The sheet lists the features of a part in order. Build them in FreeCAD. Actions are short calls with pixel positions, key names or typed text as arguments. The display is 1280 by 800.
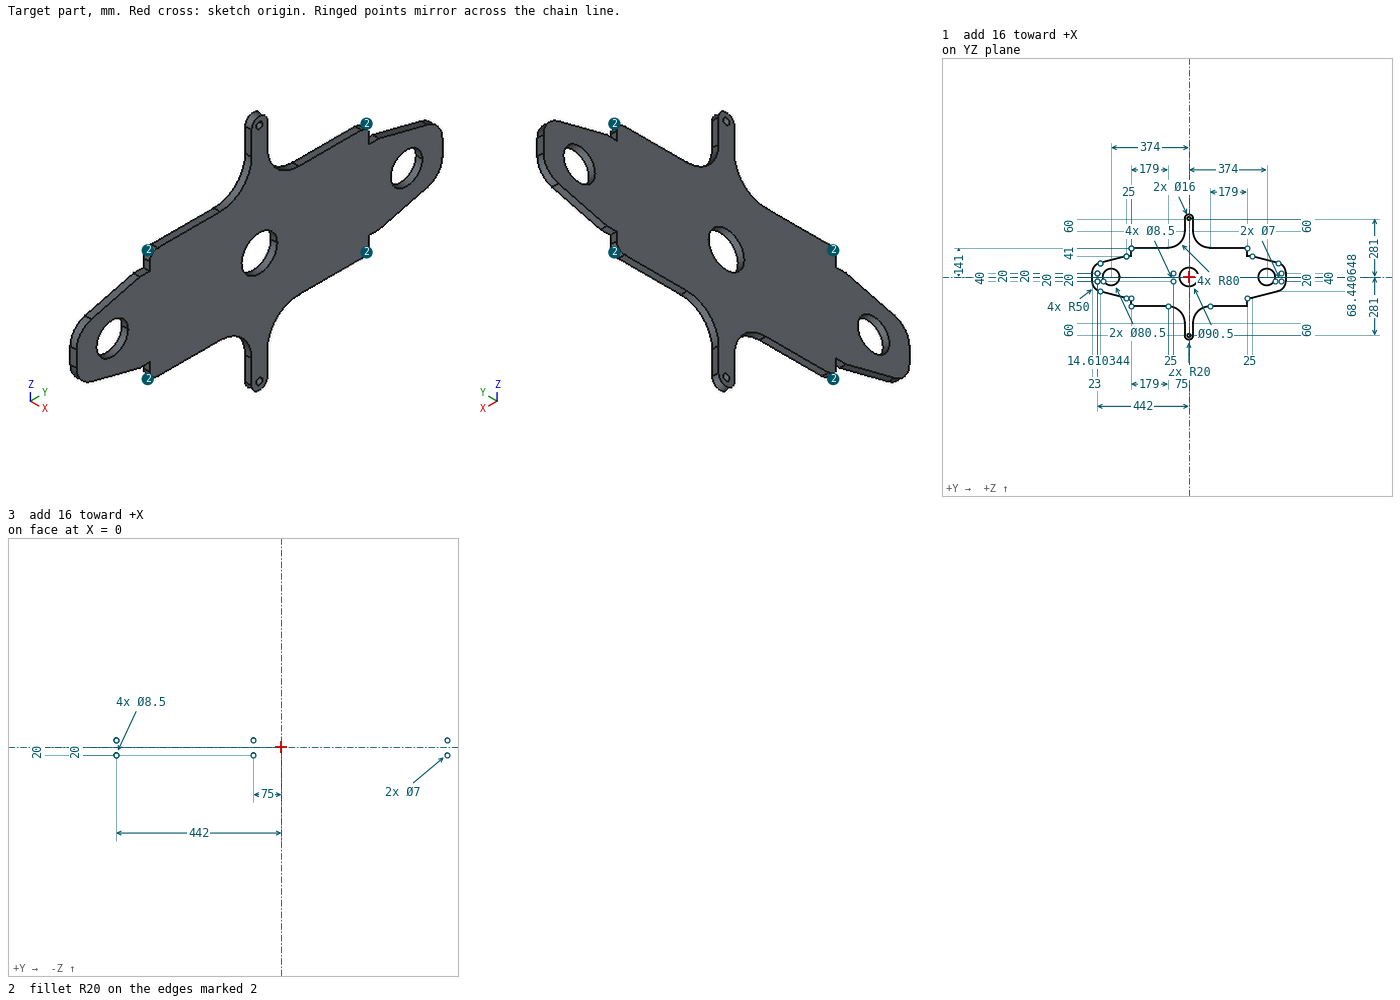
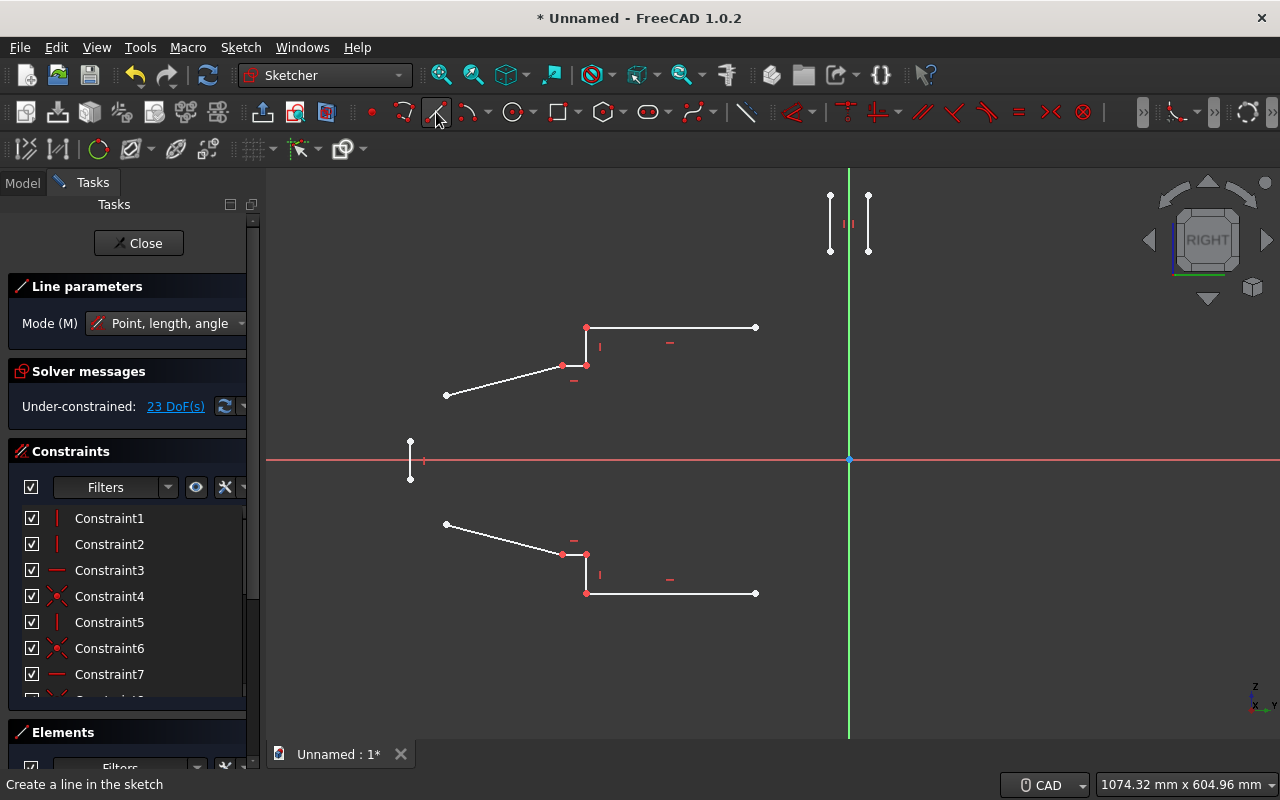
click(831, 668)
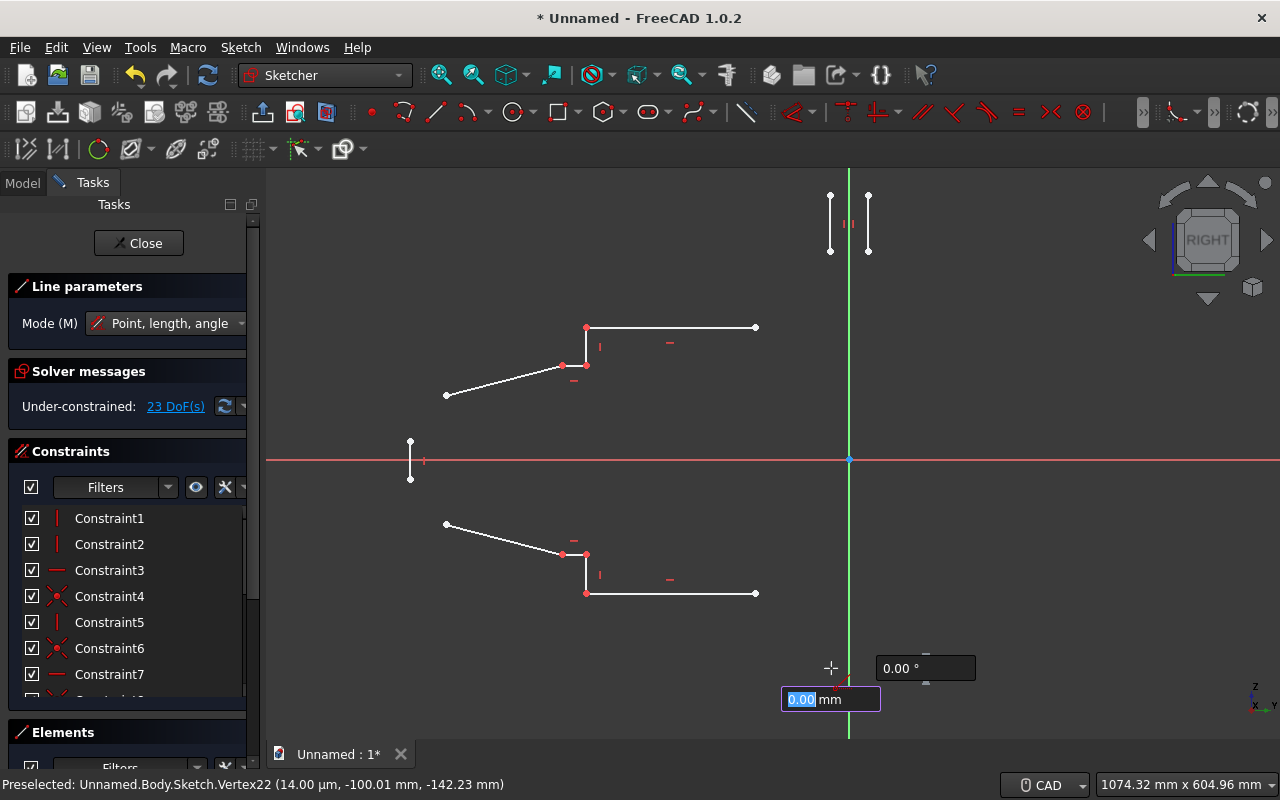
scroll(410, 441, down, 2)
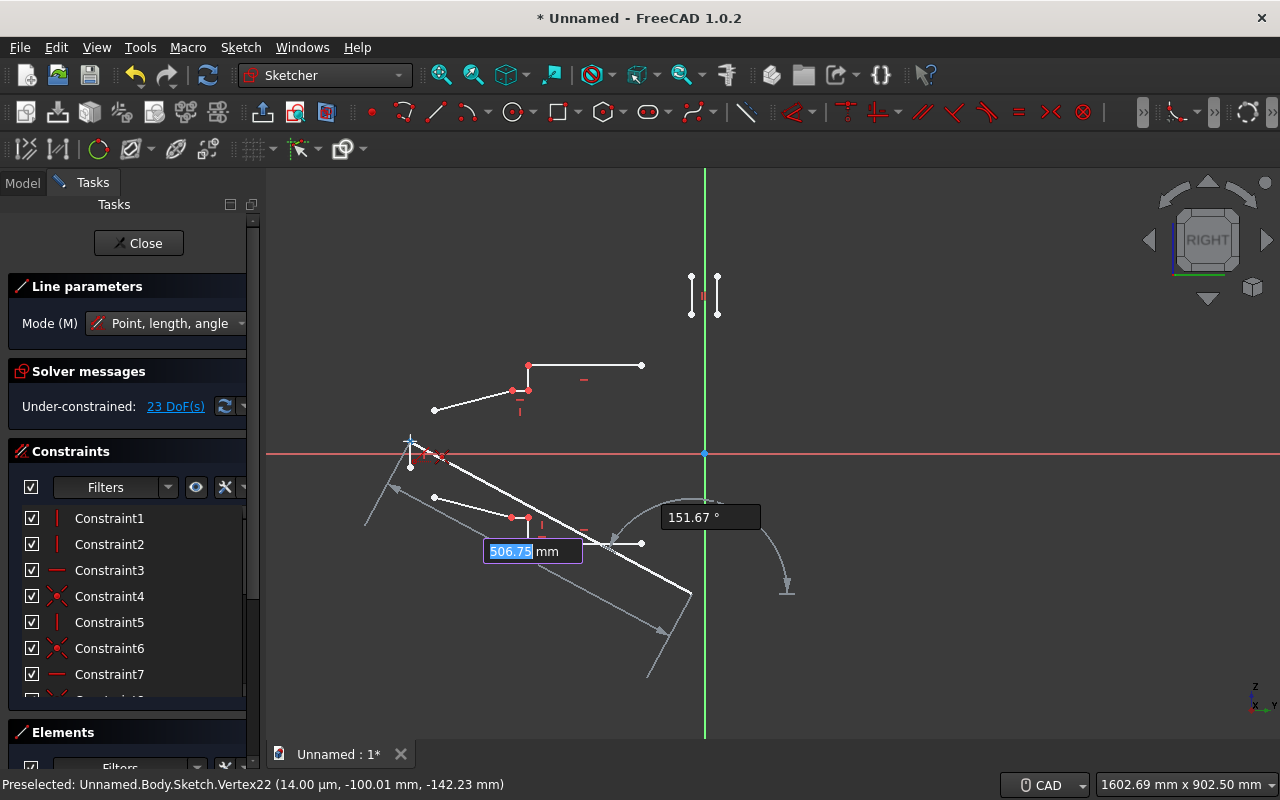
scroll(692, 632, up, 2)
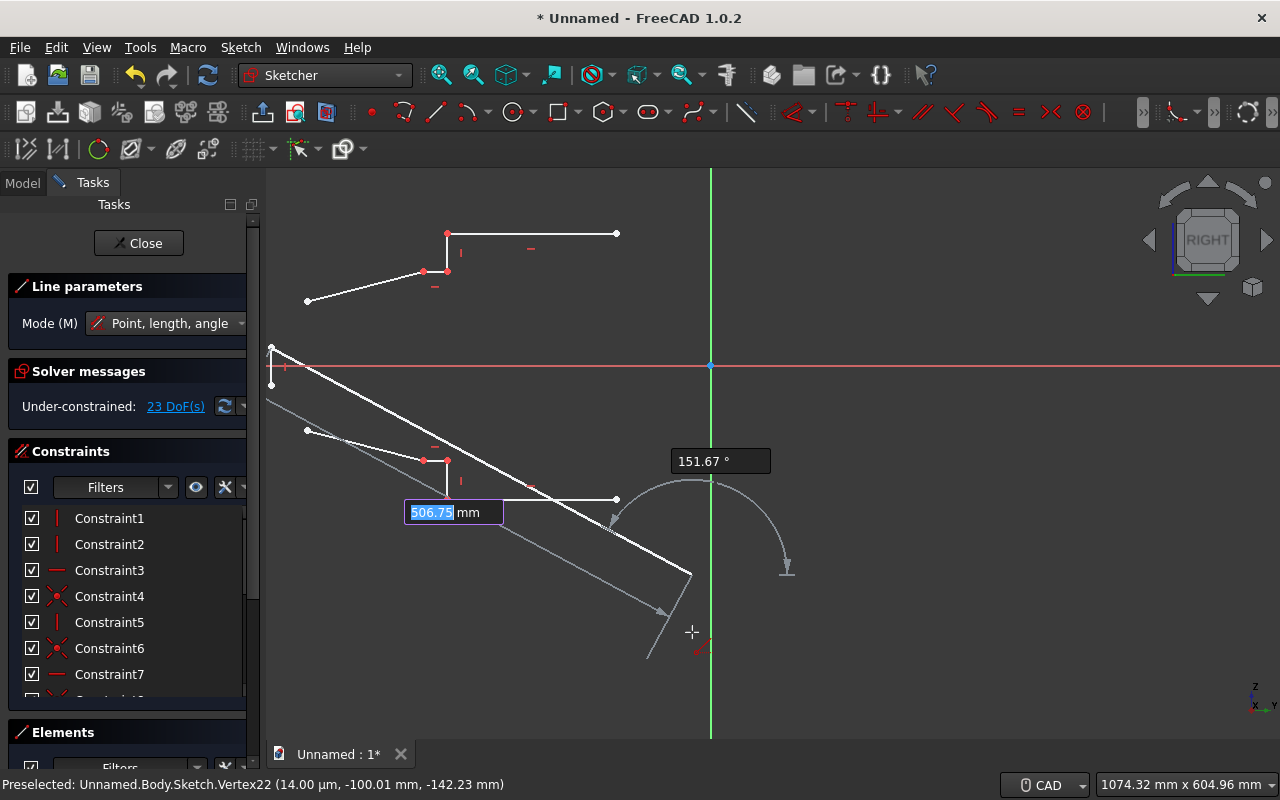
click(692, 631)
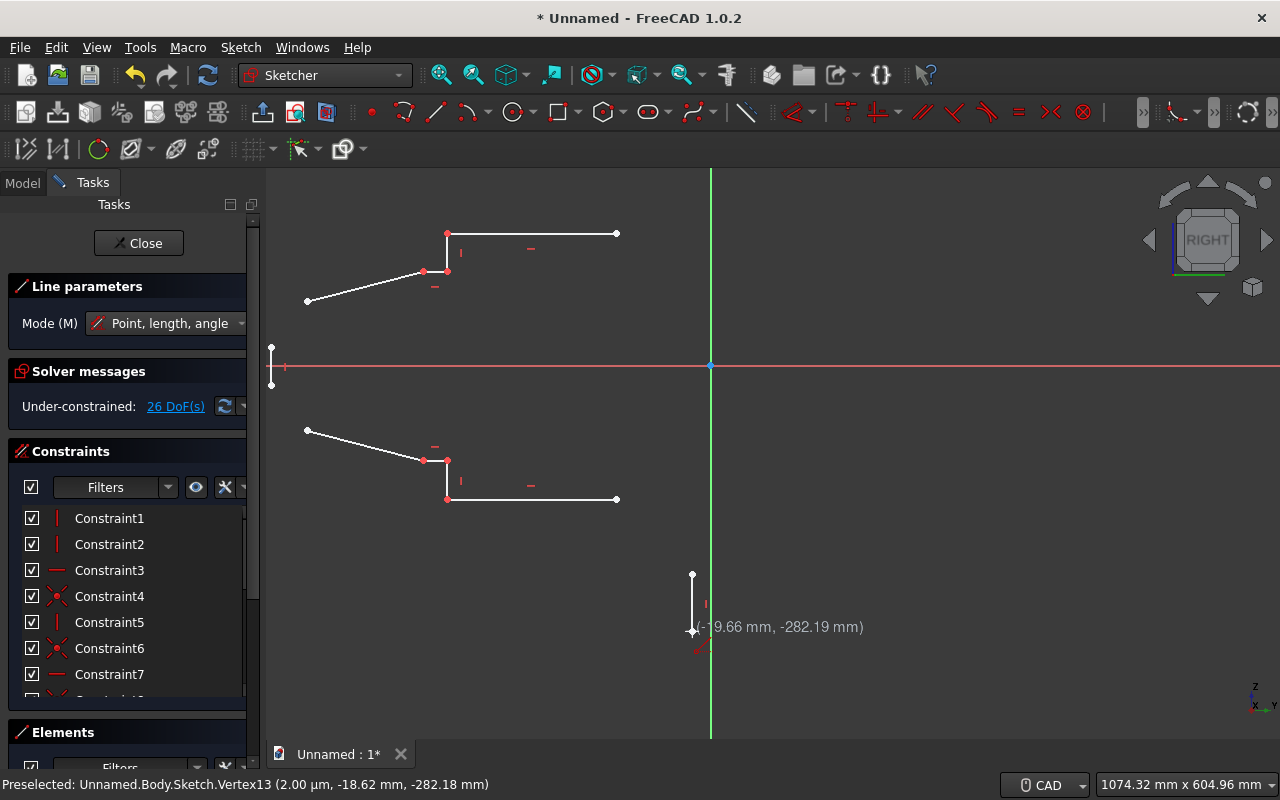
click(729, 631)
click(729, 574)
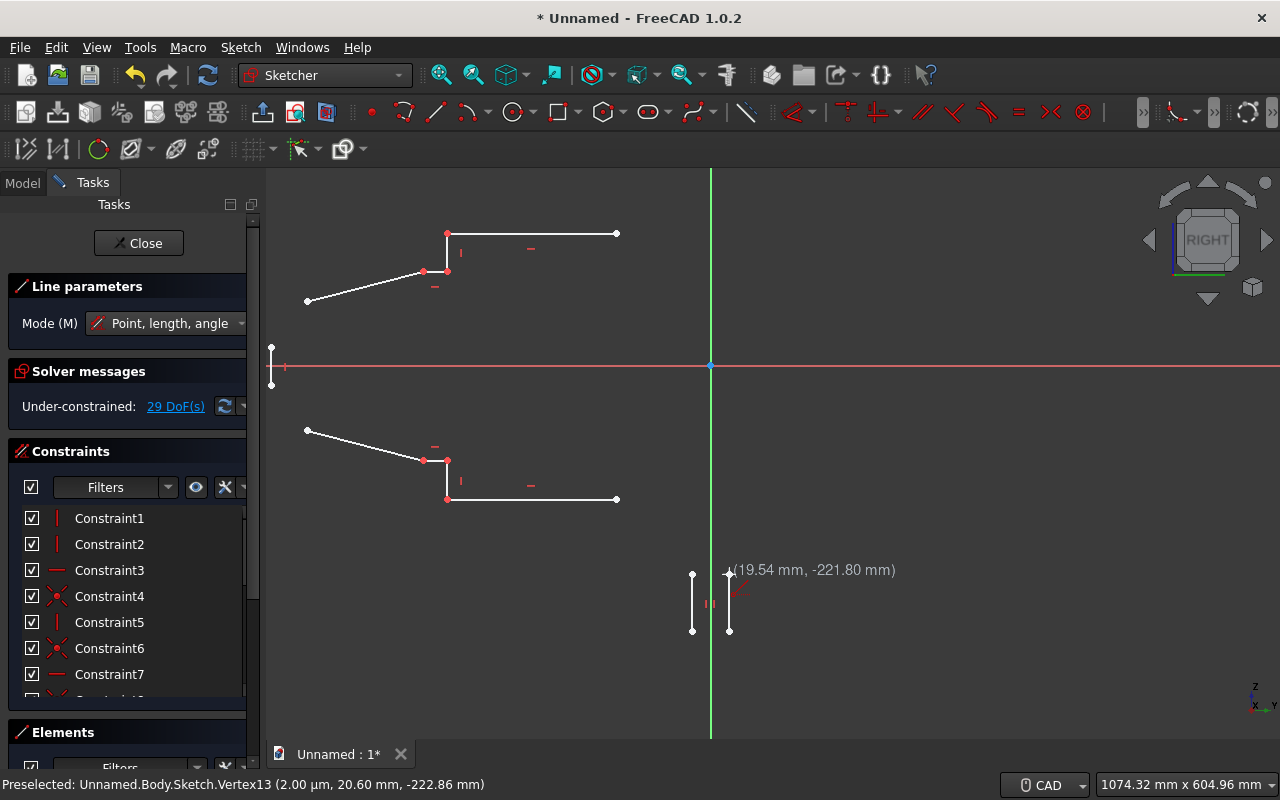
click(404, 112)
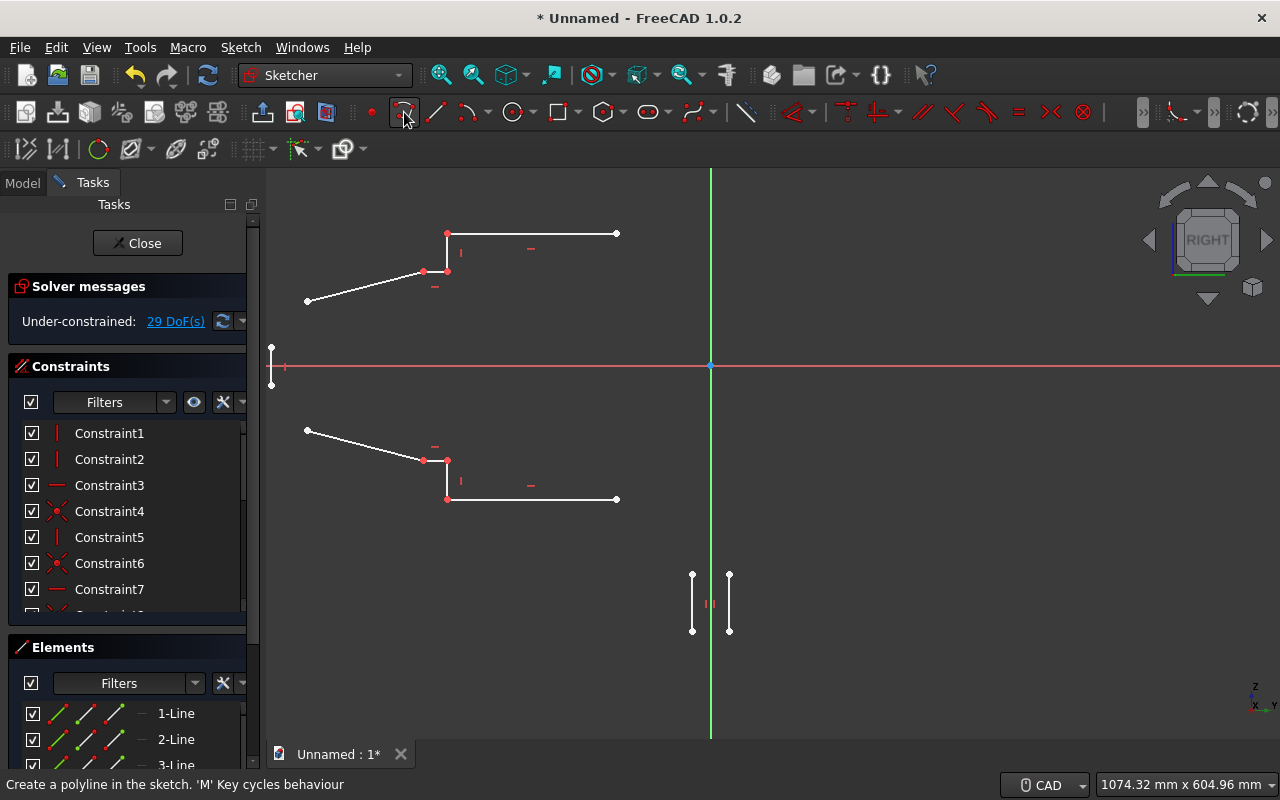
click(805, 499)
click(974, 499)
click(974, 460)
click(997, 460)
click(1114, 430)
right_click(1114, 430)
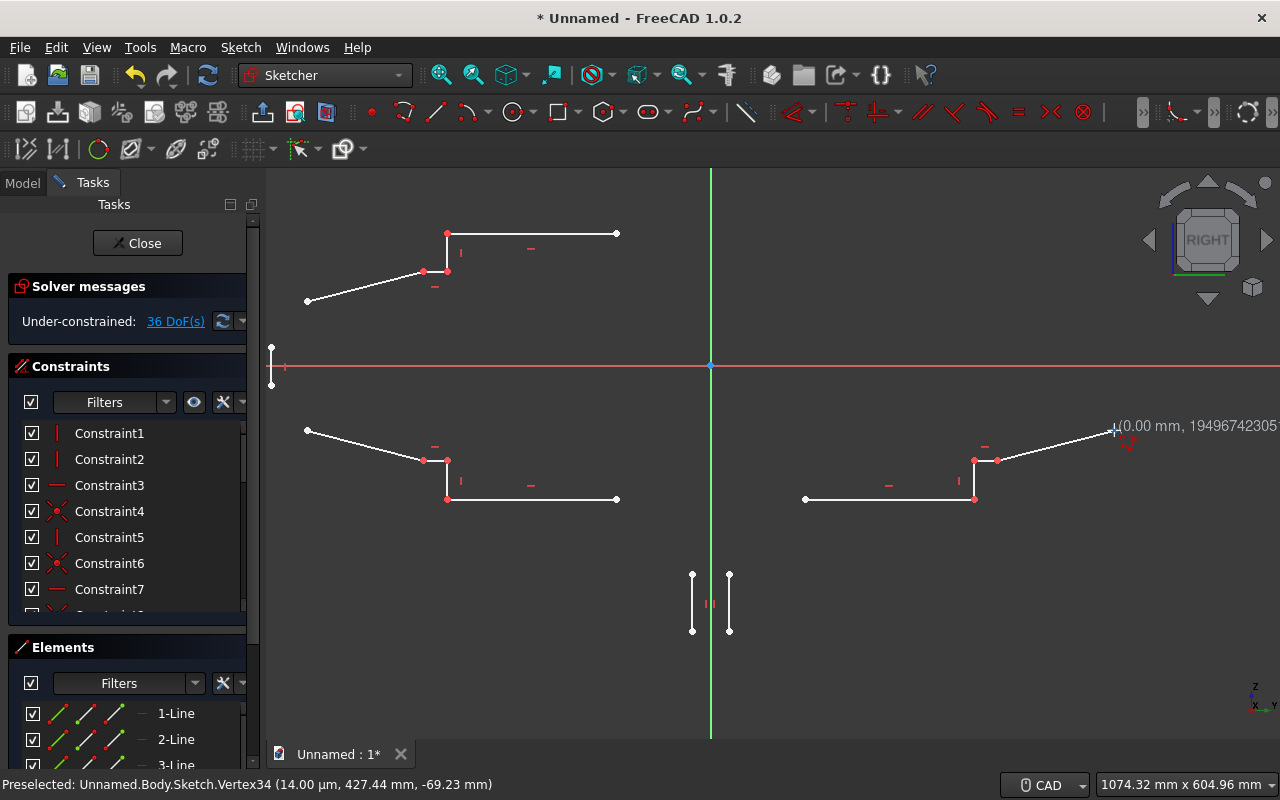
click(436, 112)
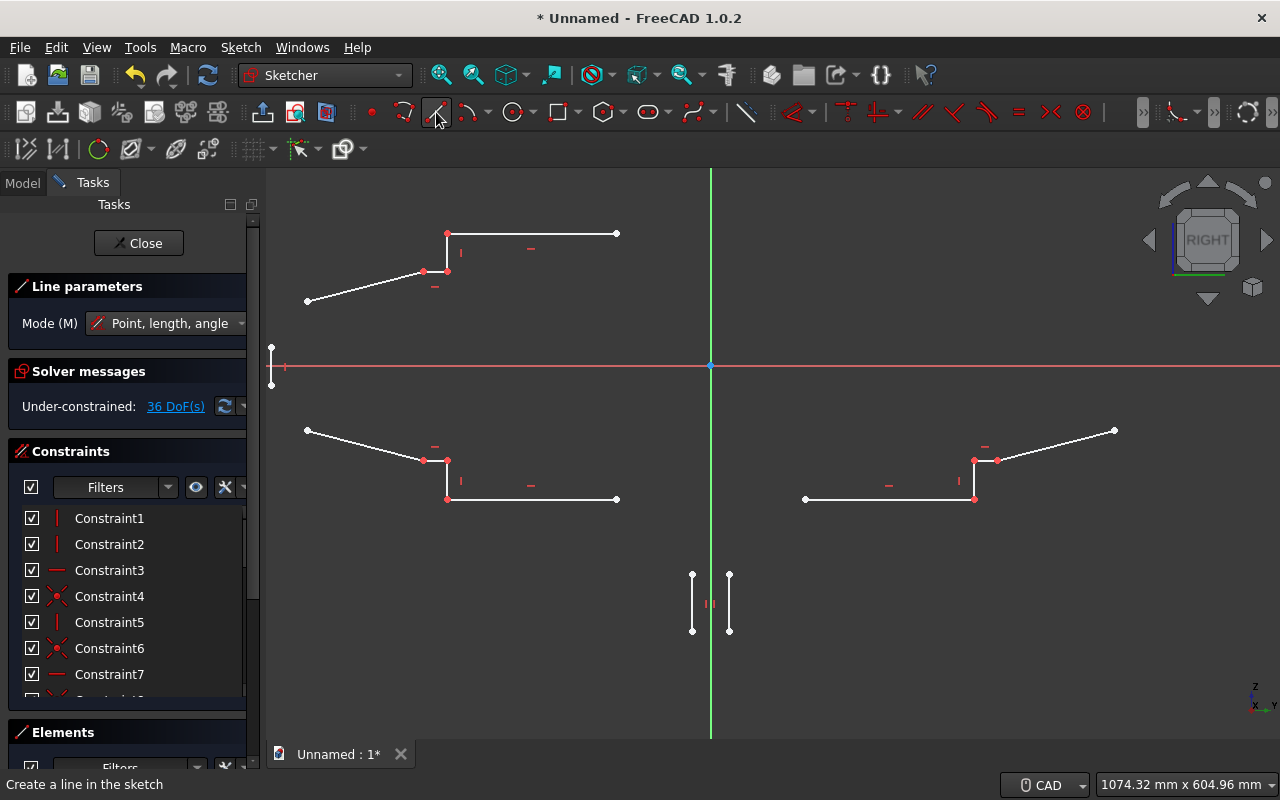
scroll(692, 632, down, 2)